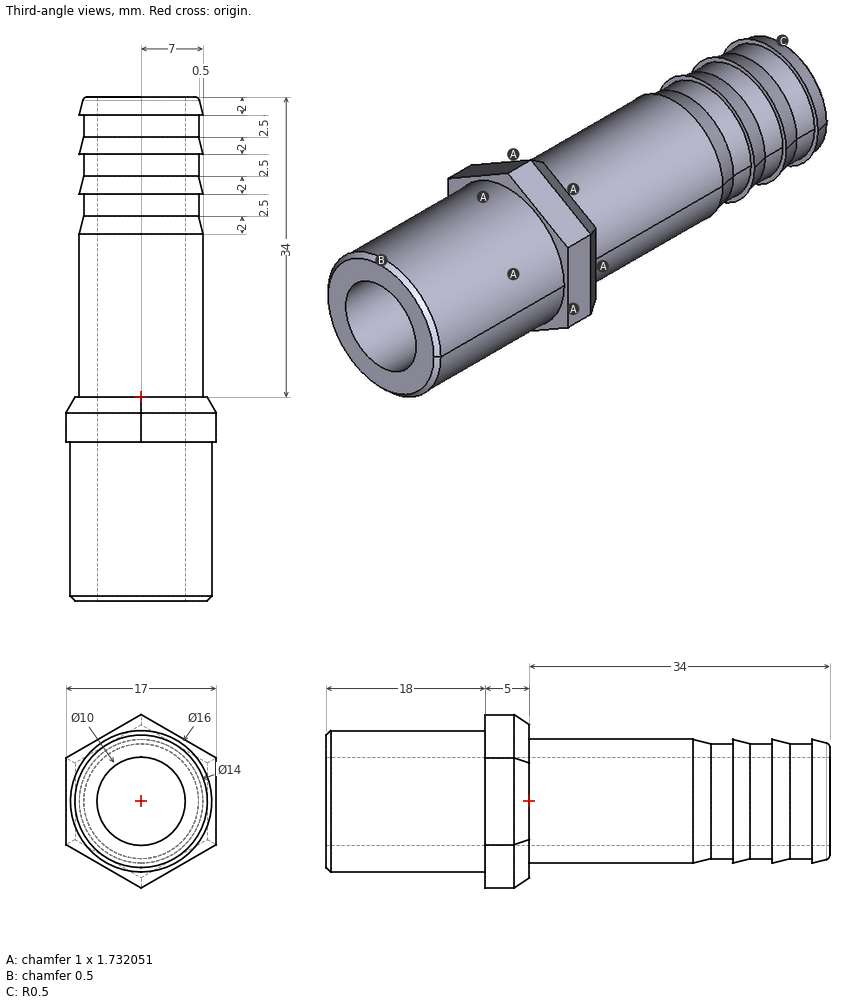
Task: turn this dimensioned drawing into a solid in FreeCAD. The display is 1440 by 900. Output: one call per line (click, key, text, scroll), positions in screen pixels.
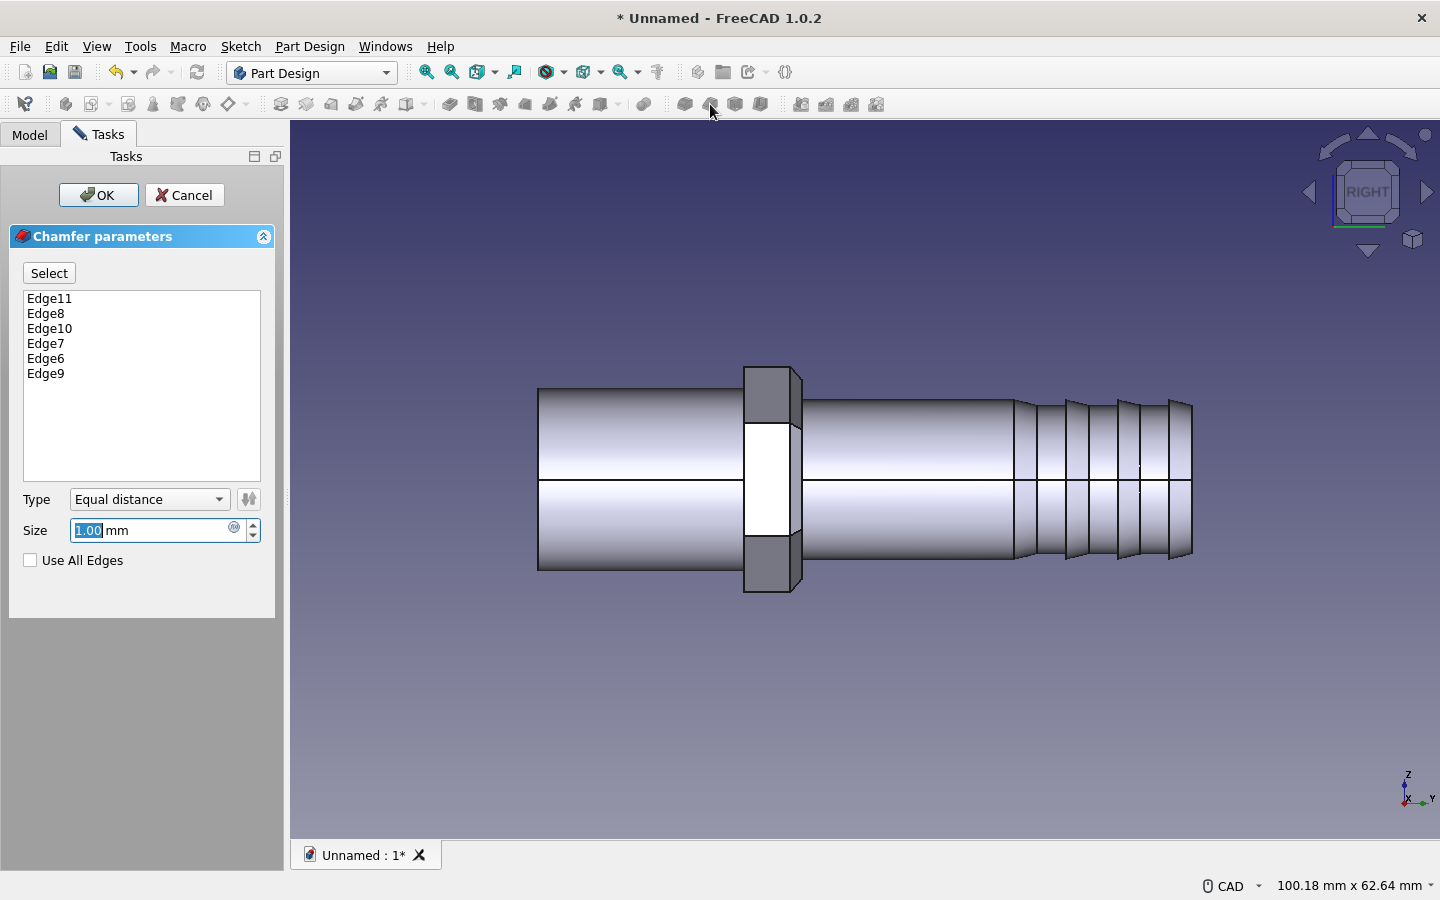
text(1)
key(Tab)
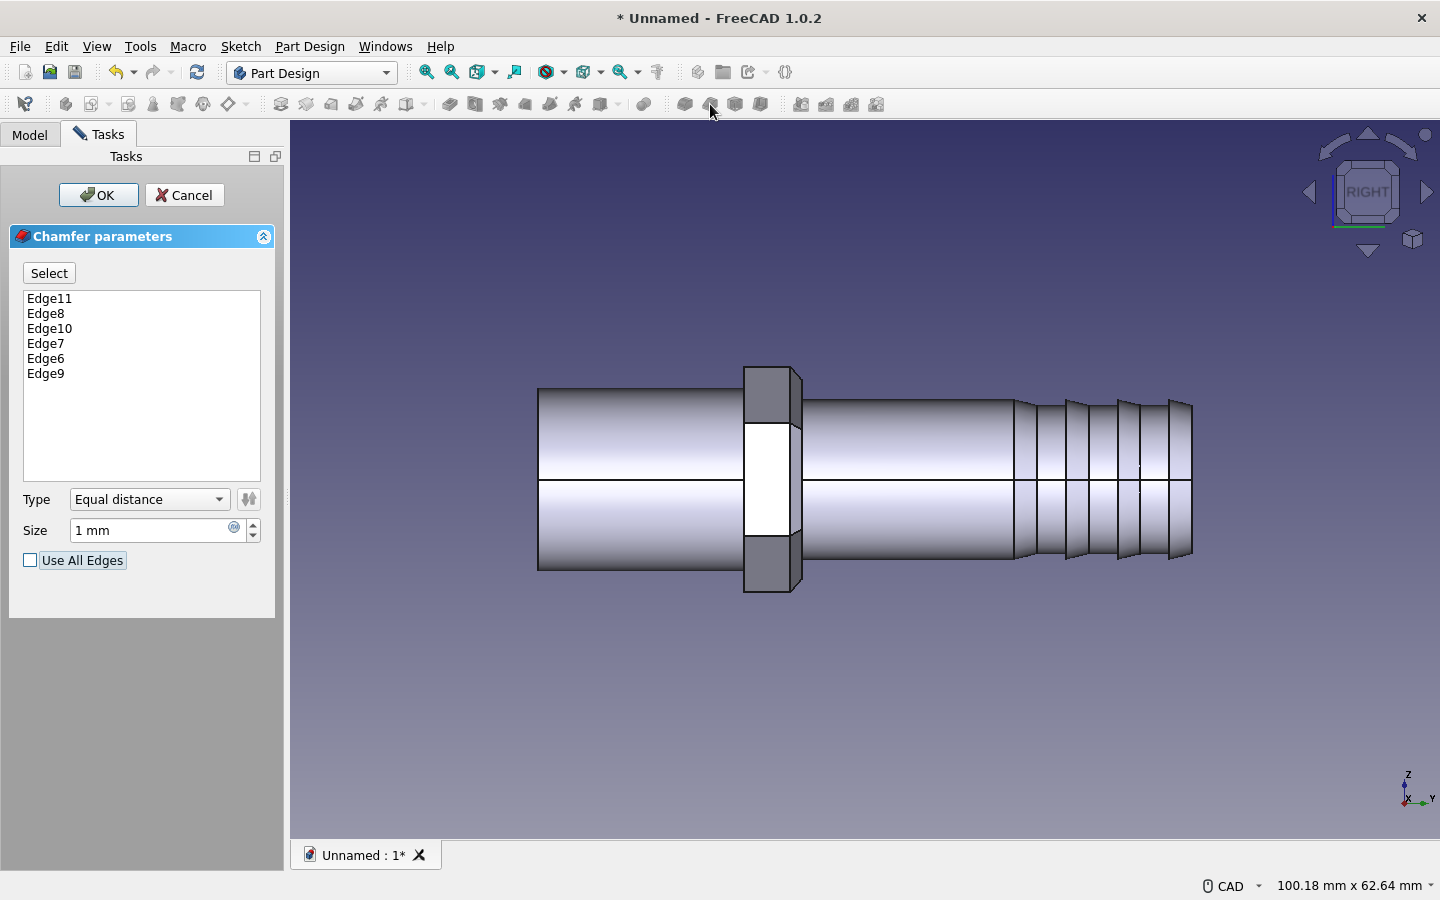
click(150, 500)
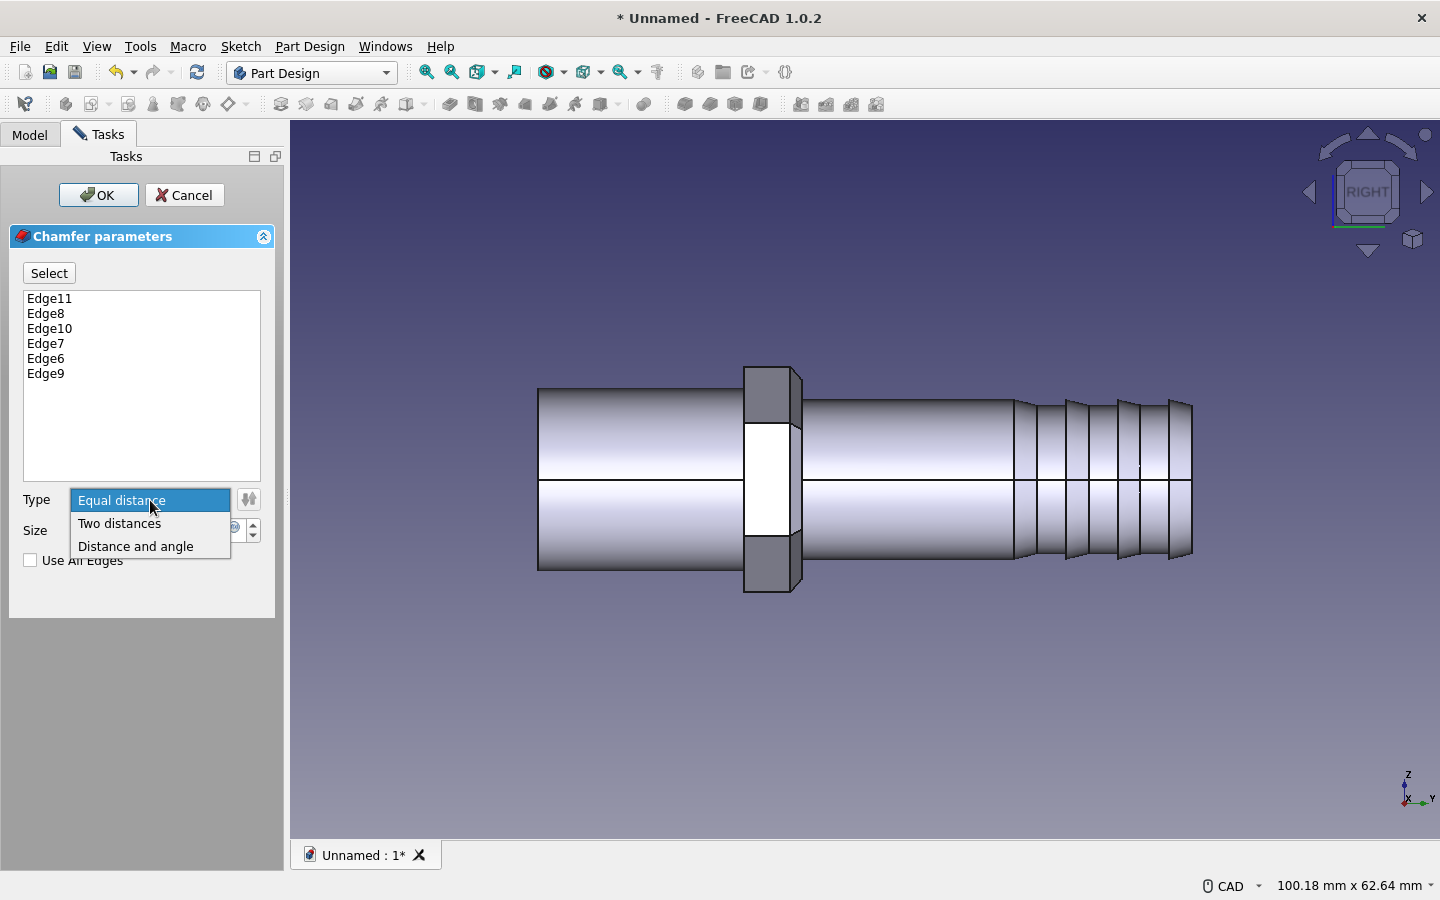
click(148, 524)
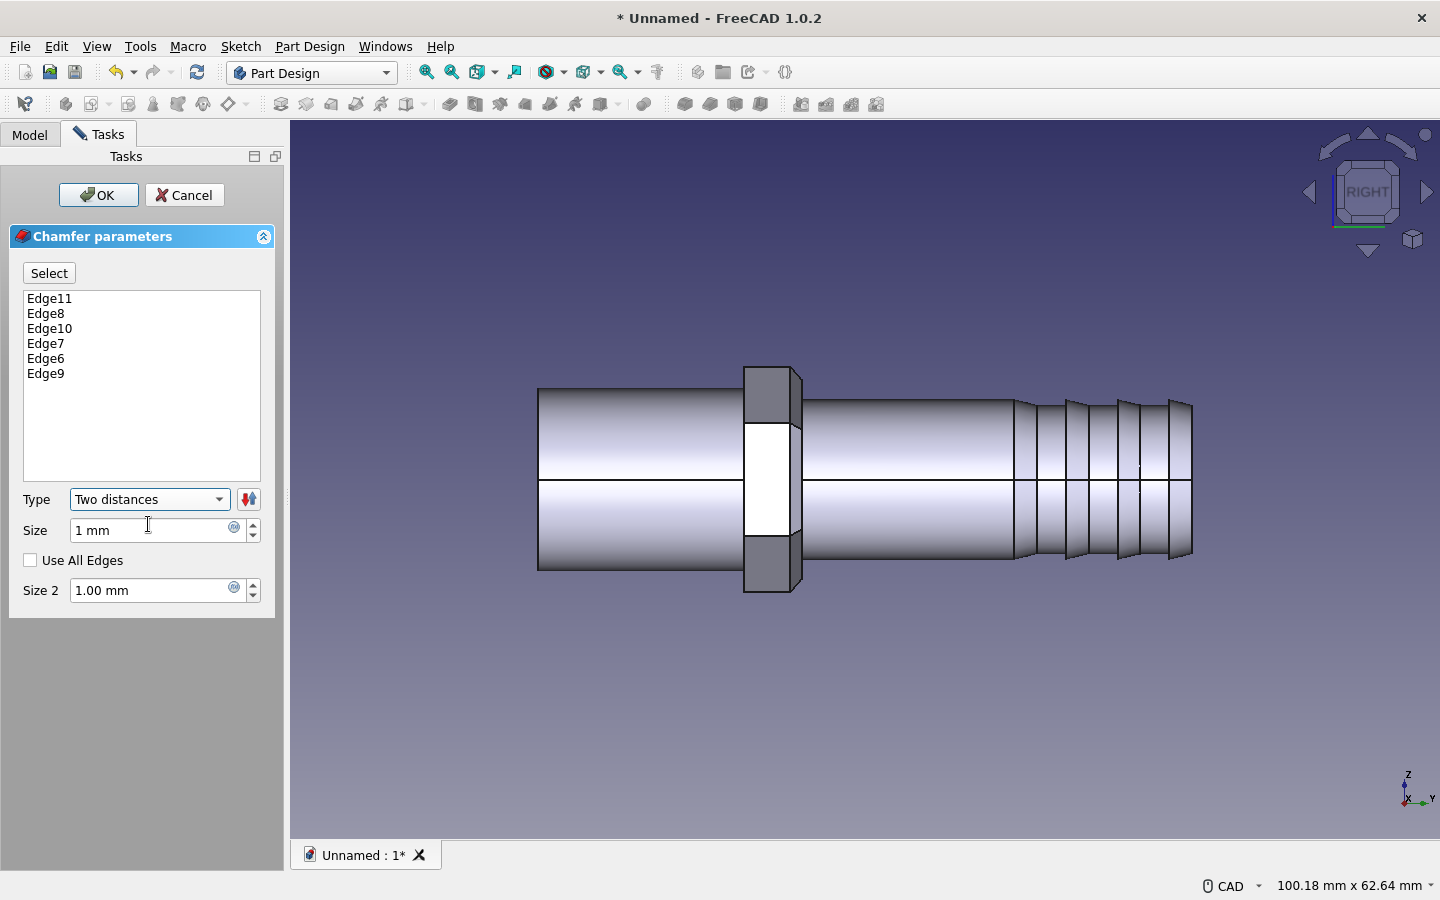
triple_click(158, 590)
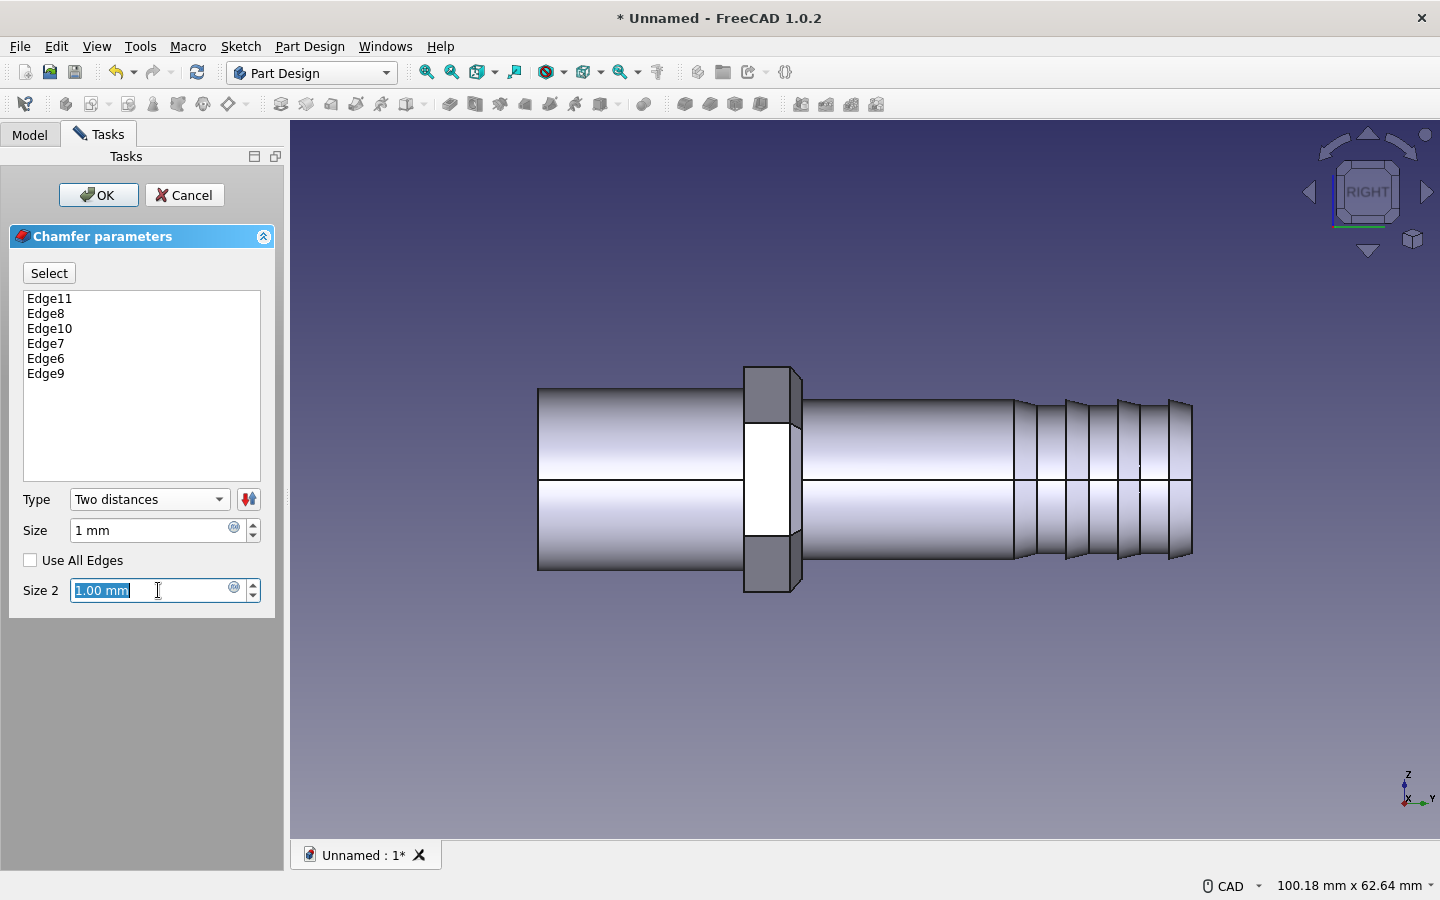
text(1.732051)
key(Tab)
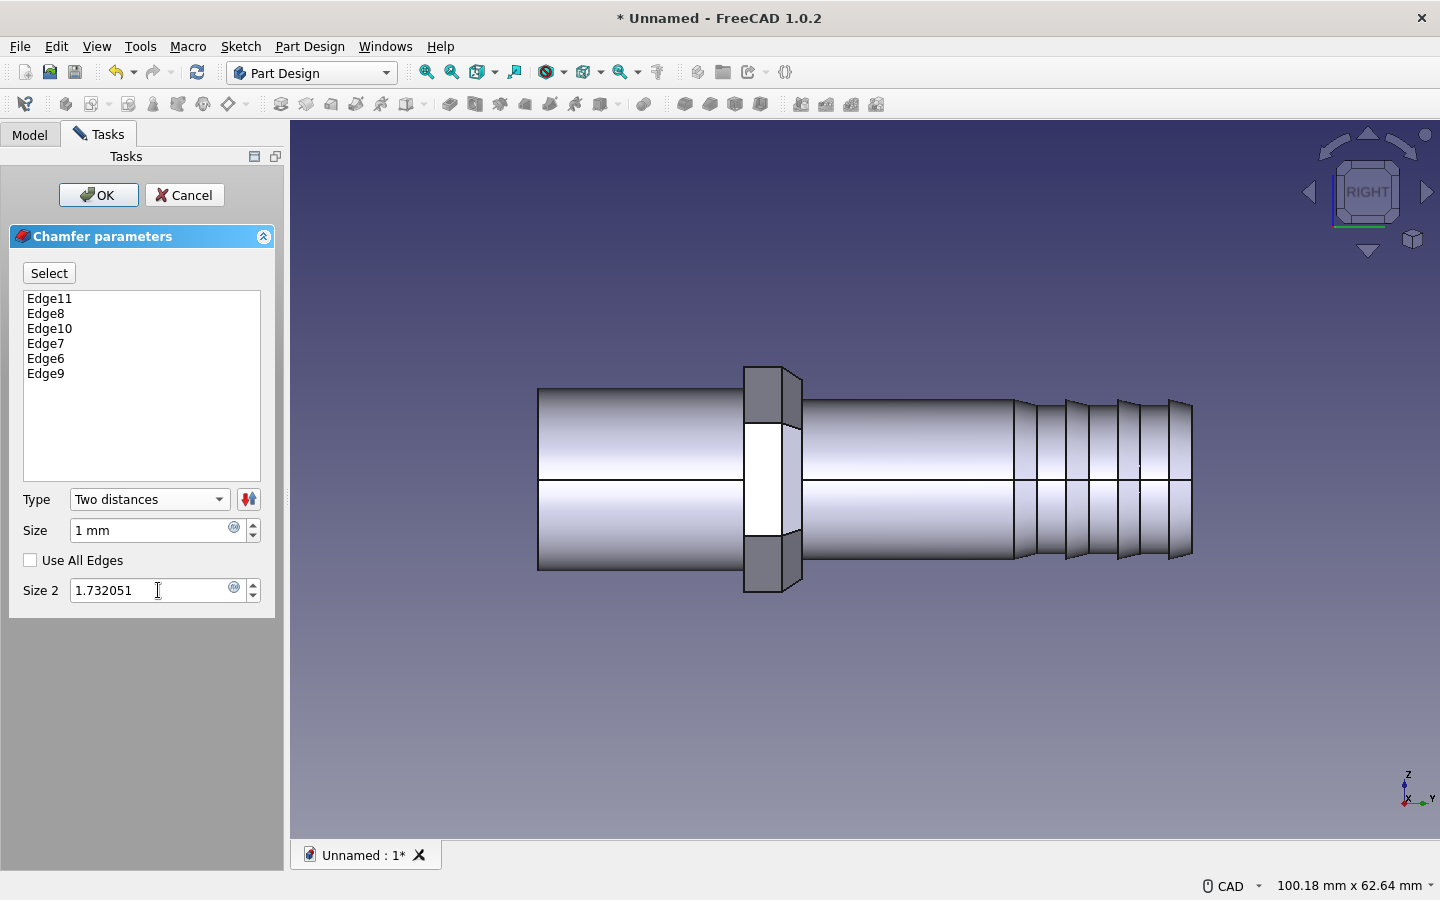
click(99, 195)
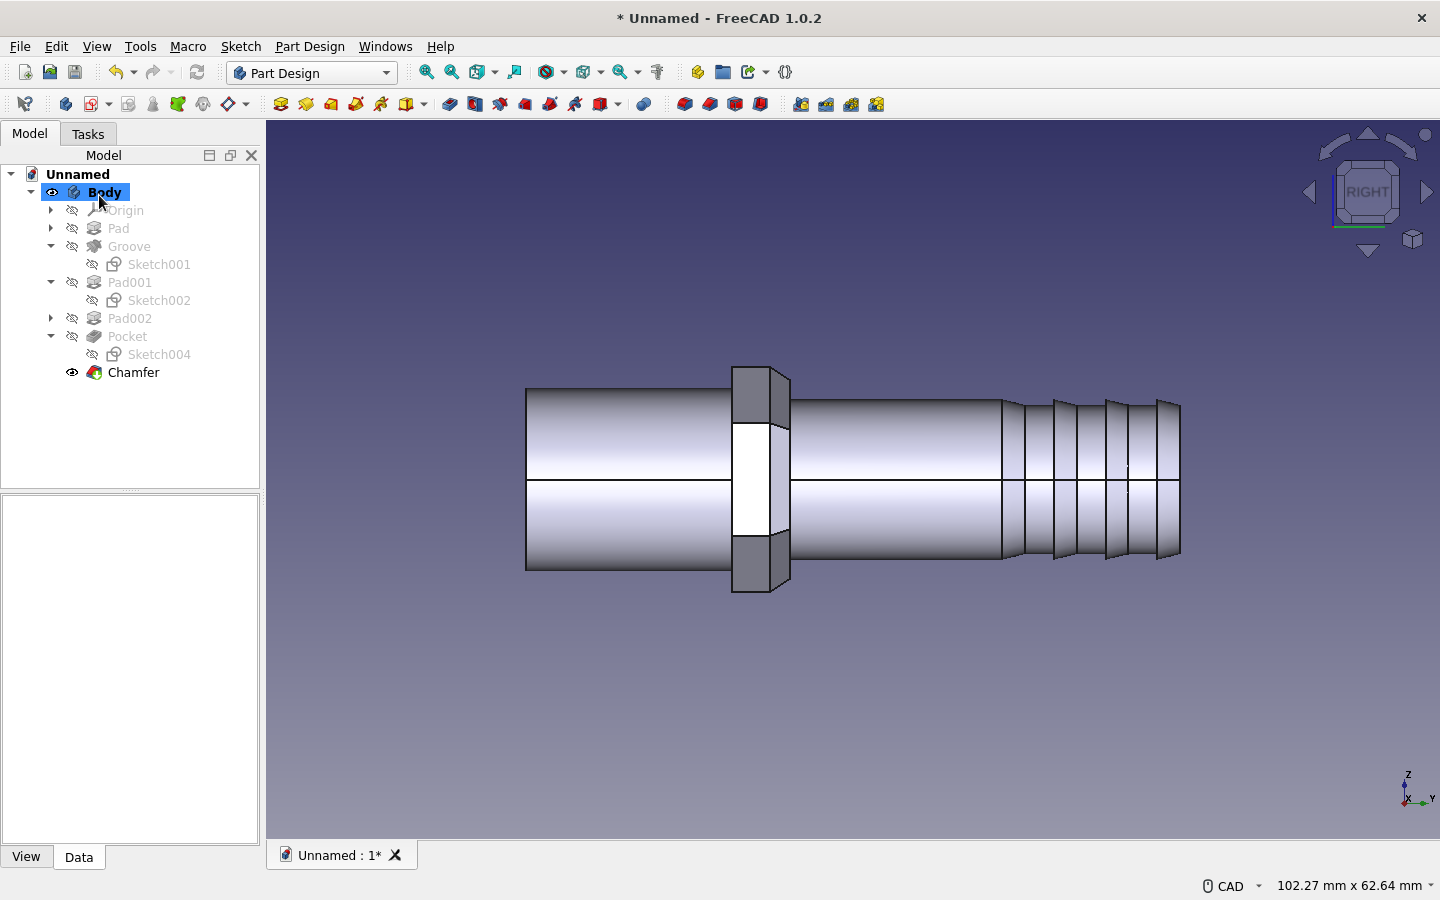
click(526, 425)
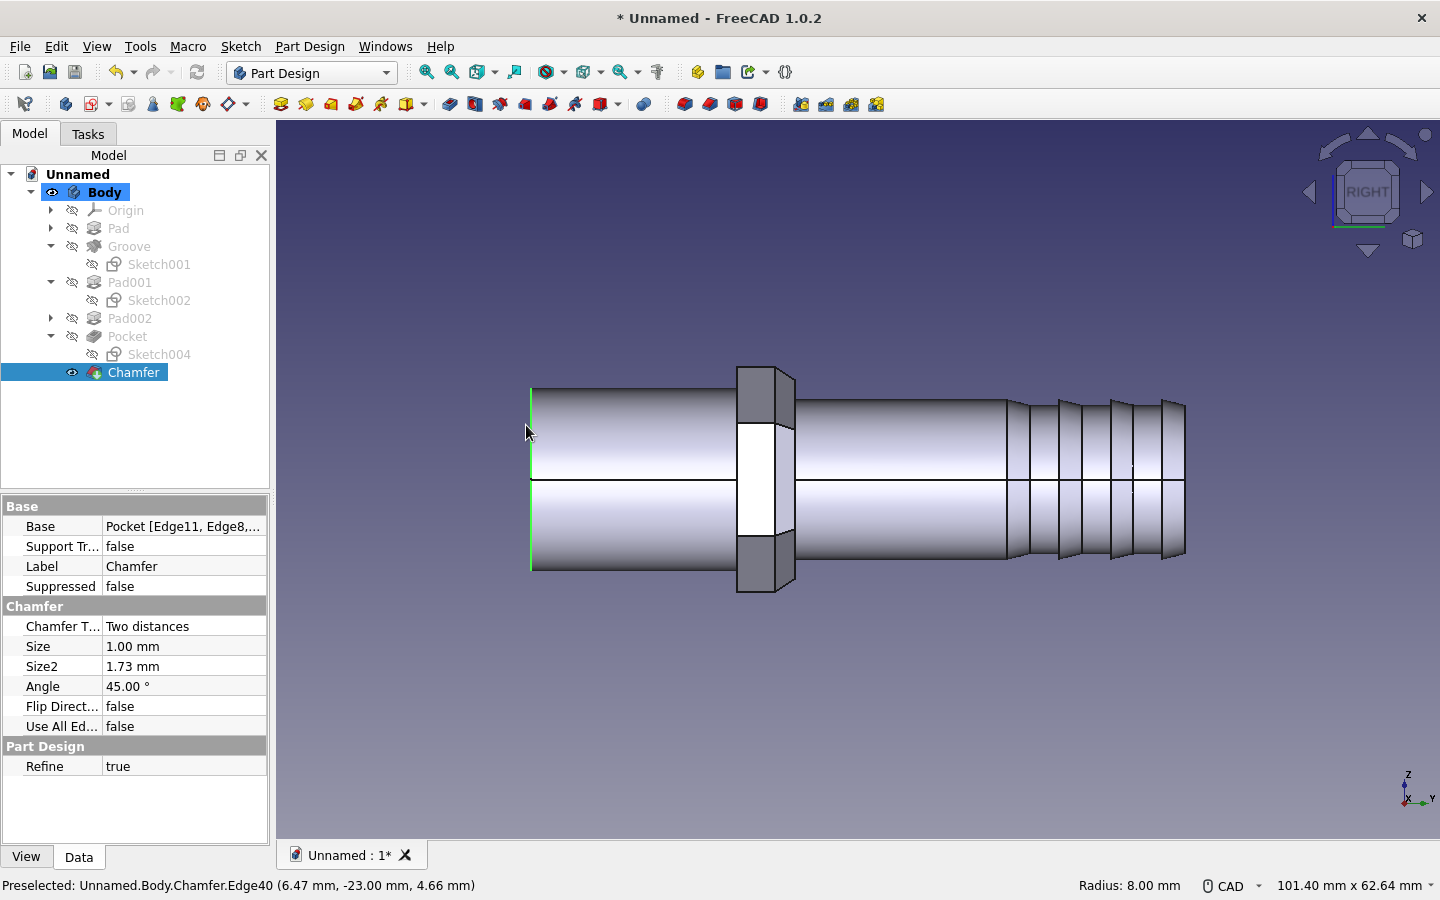
click(710, 104)